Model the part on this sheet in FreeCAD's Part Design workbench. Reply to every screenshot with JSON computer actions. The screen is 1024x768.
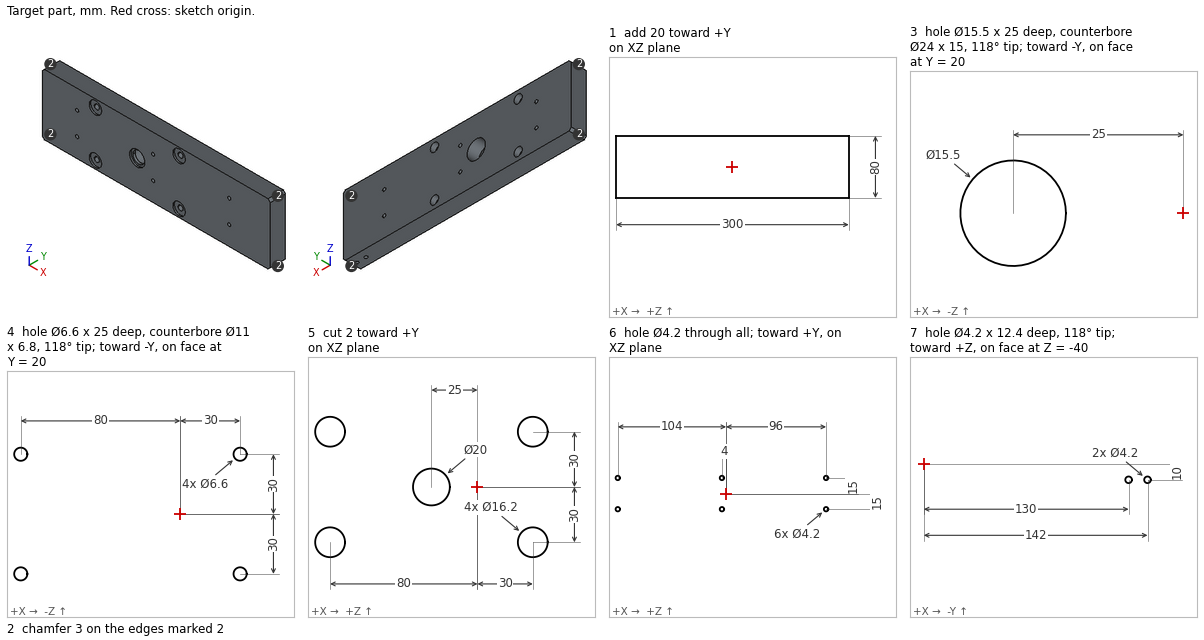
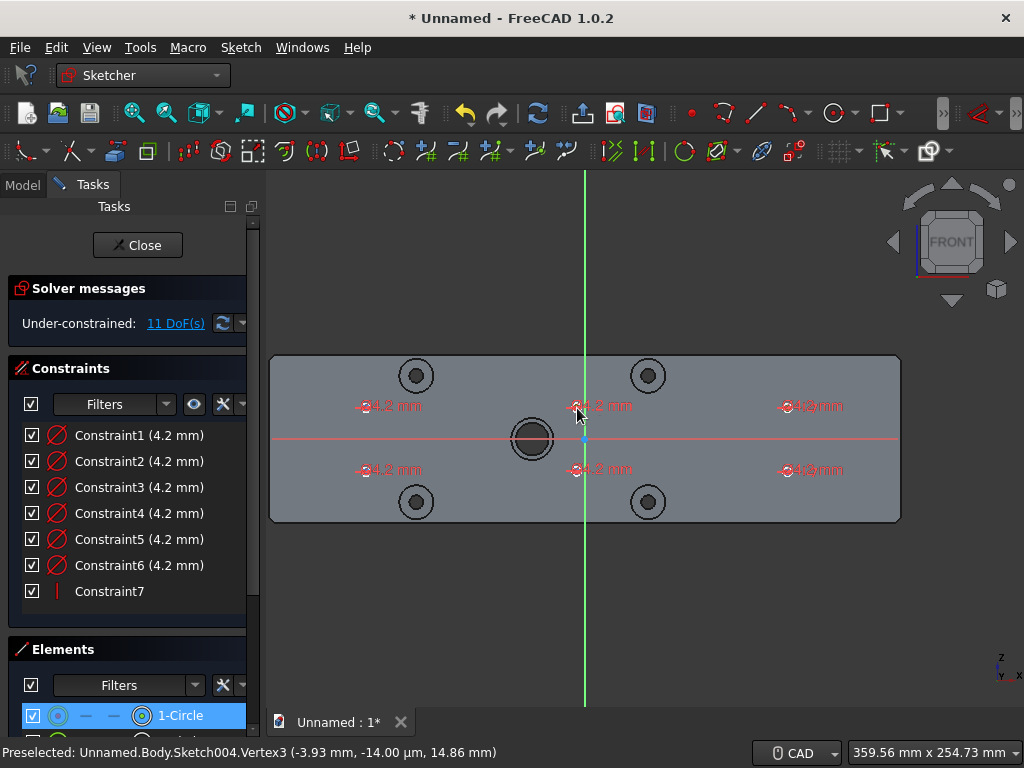
{"action": "key", "text": "h"}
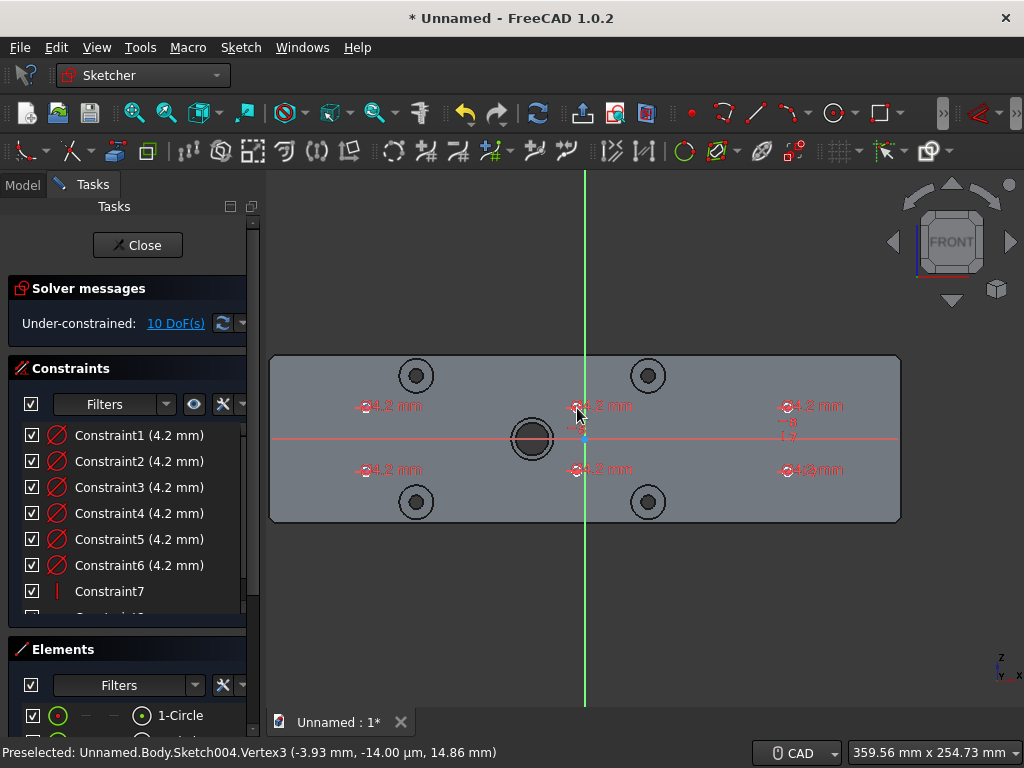
{"action": "left_click", "coordinate": [577, 408]}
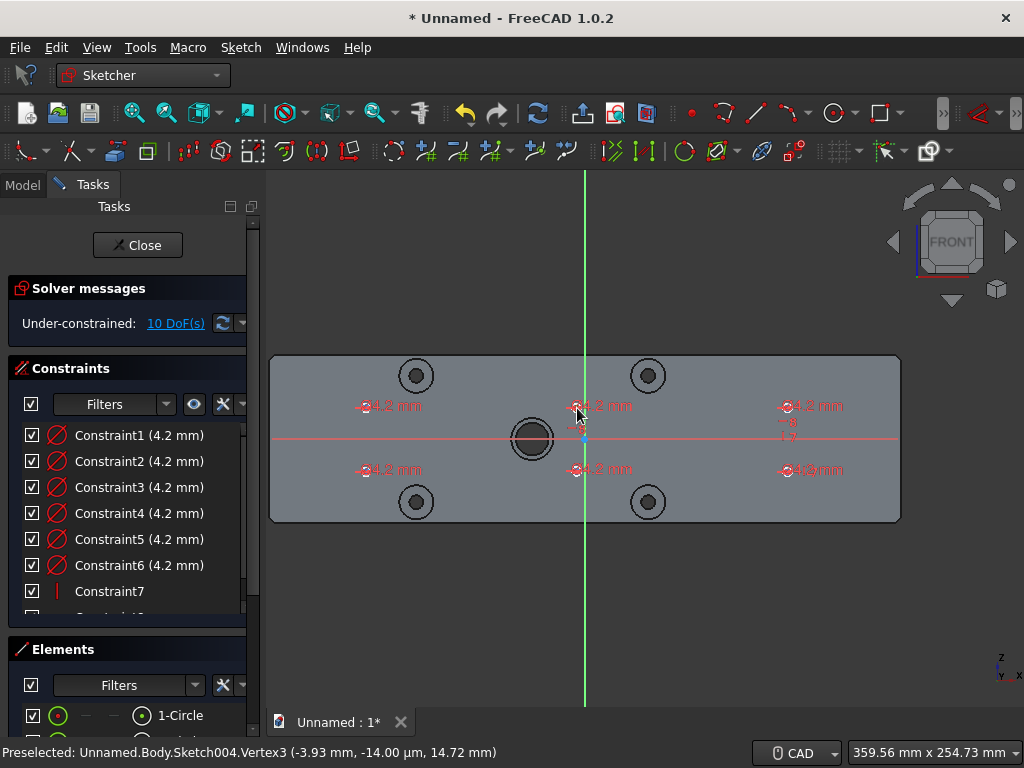
{"action": "left_click", "coordinate": [577, 471]}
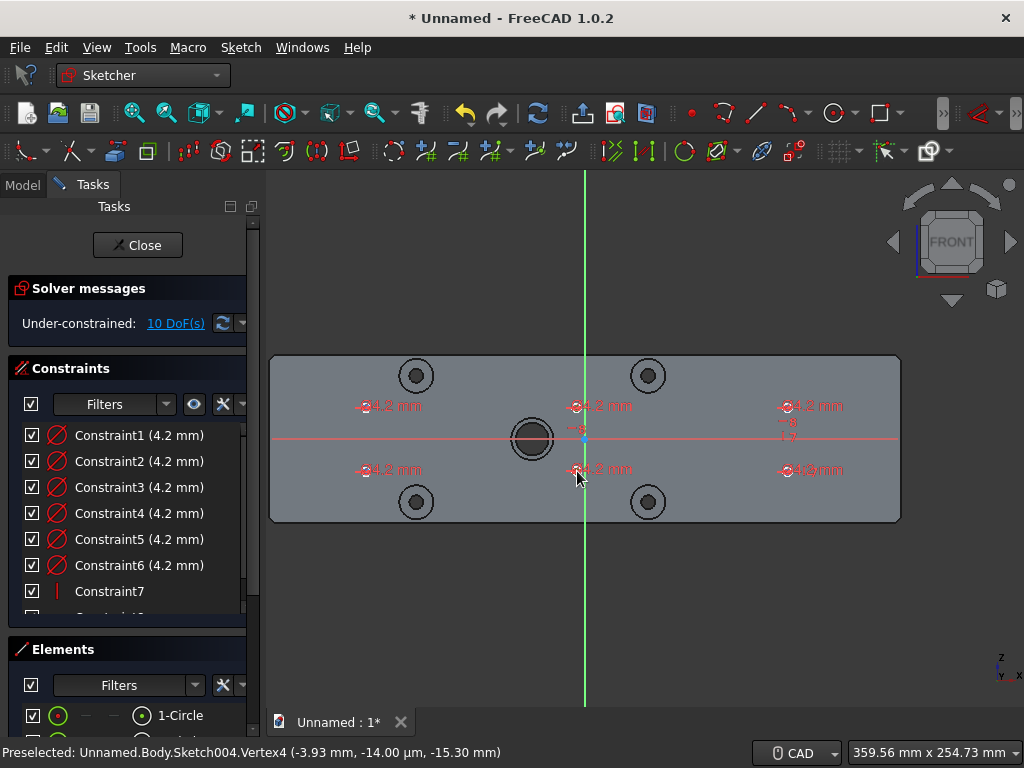
{"action": "key", "text": "v"}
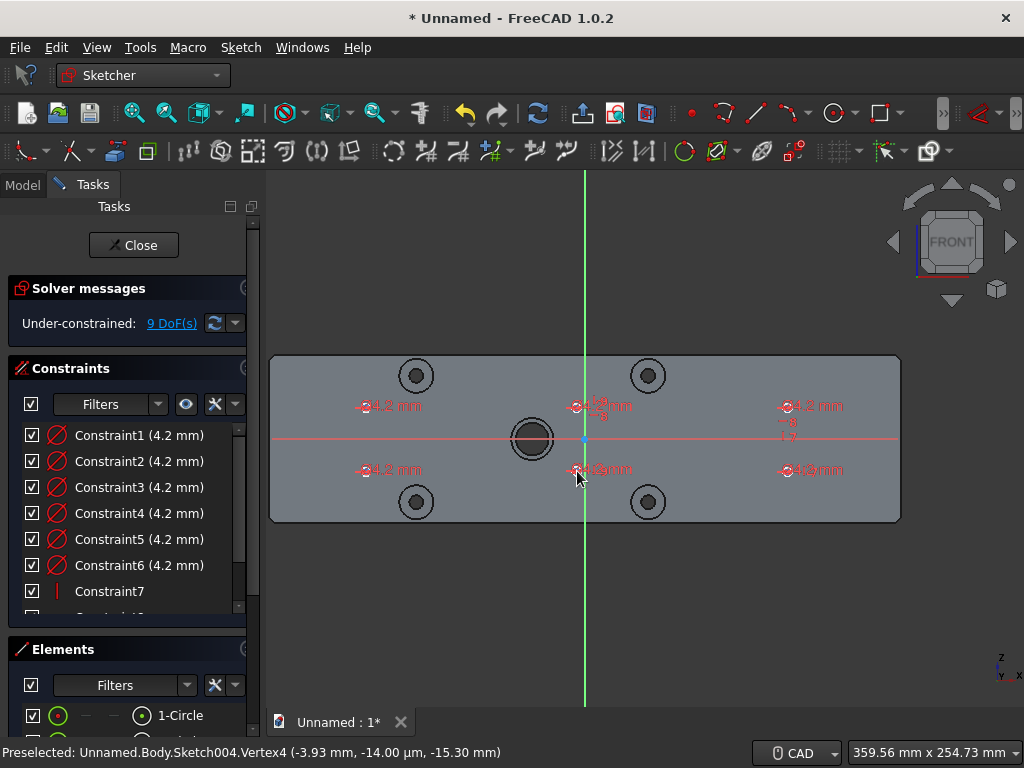
{"action": "left_click", "coordinate": [787, 472]}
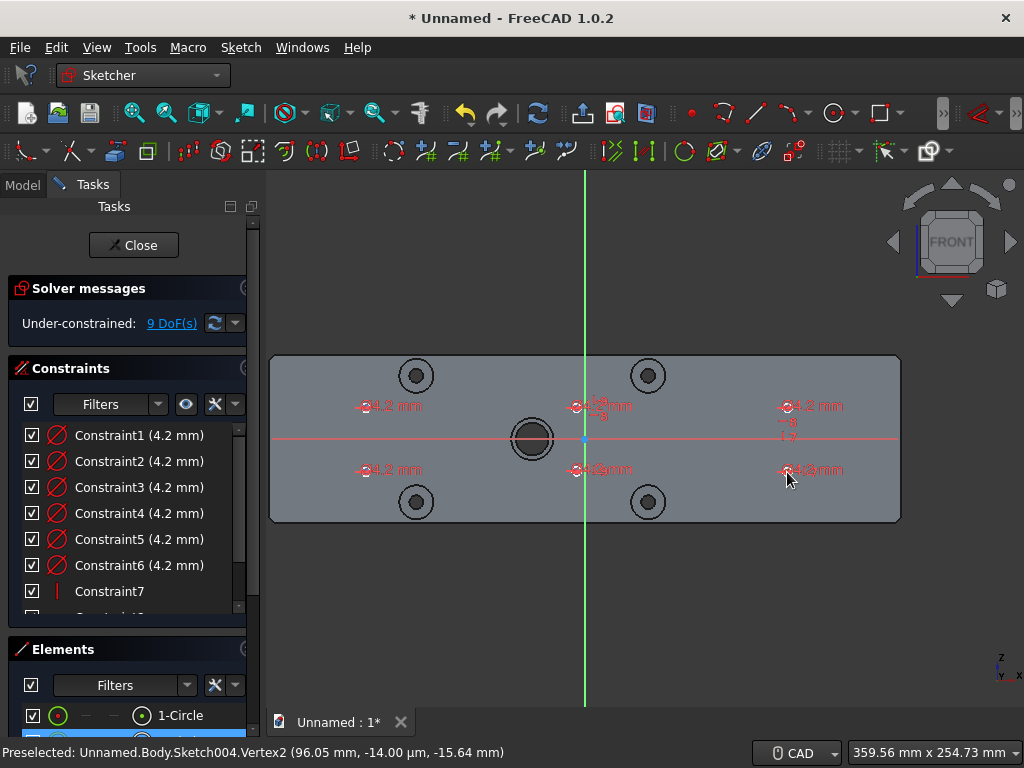
{"action": "left_click", "coordinate": [577, 471]}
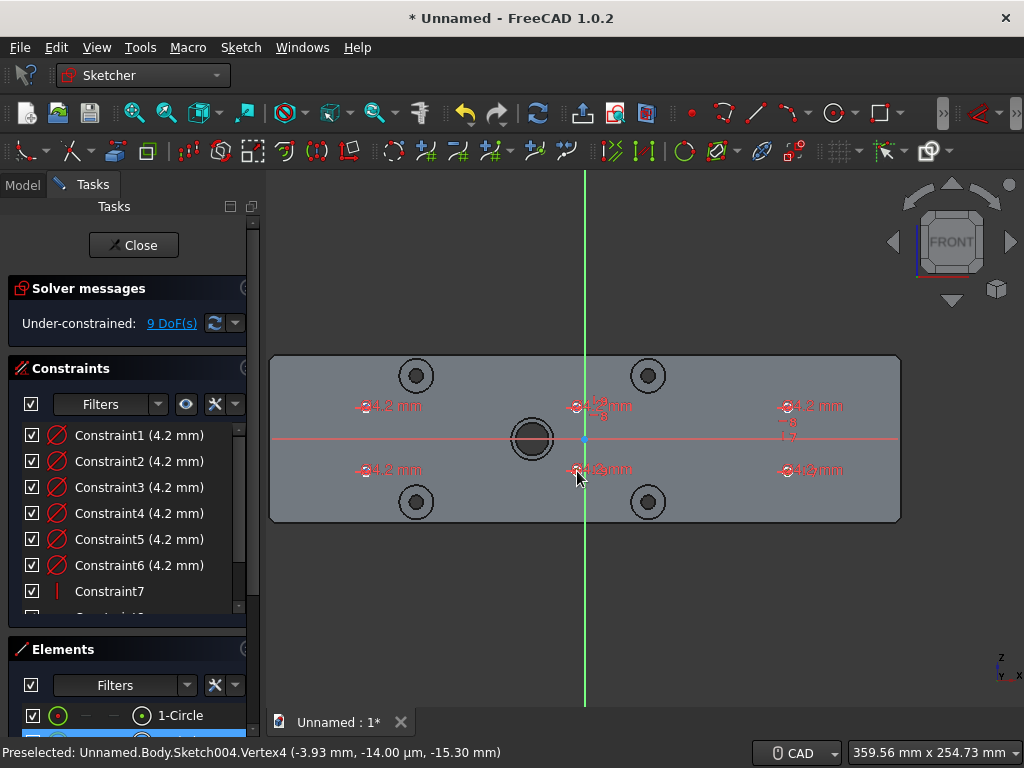
{"action": "key", "text": "h"}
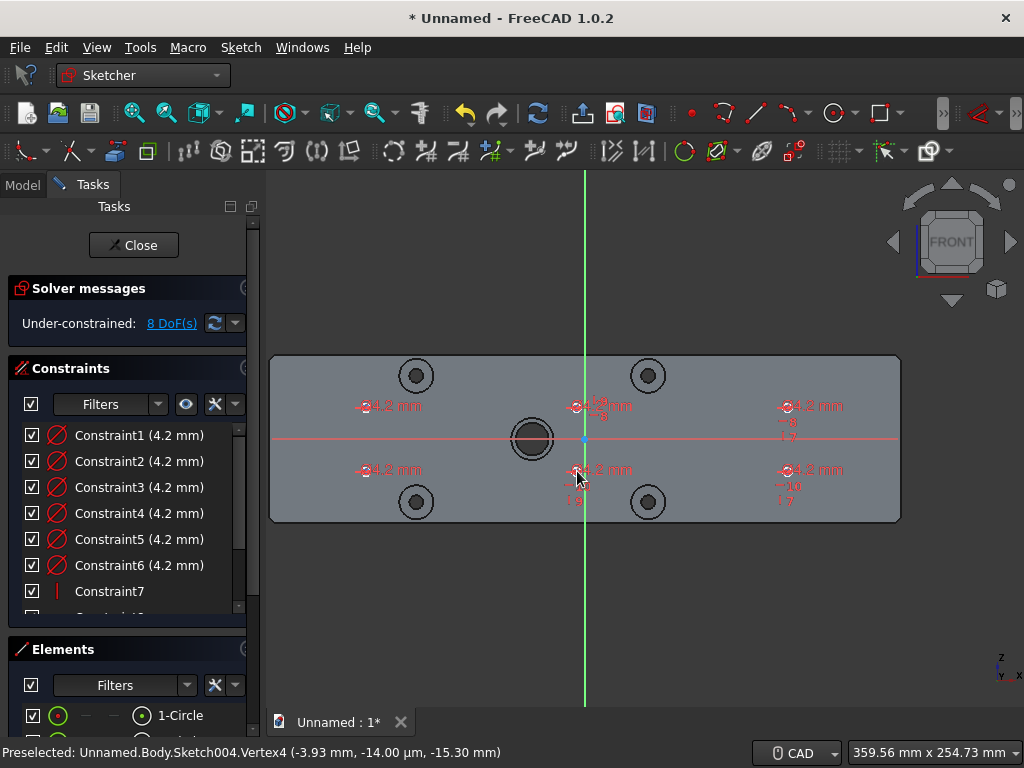
{"action": "left_click", "coordinate": [577, 408]}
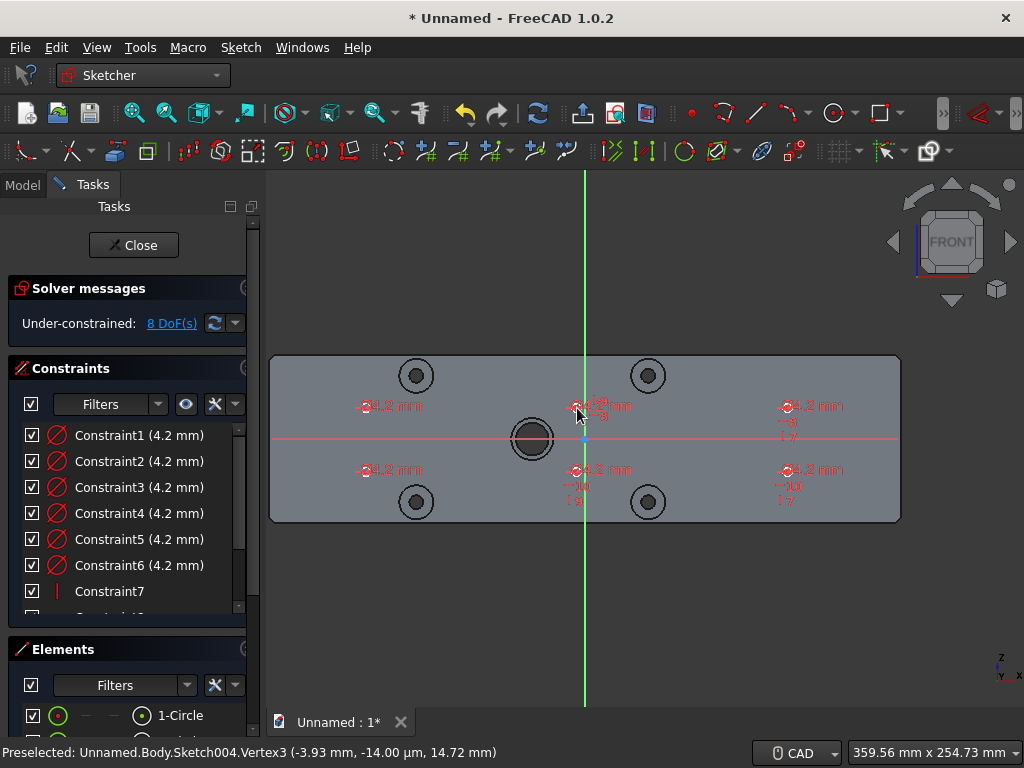
{"action": "left_click", "coordinate": [366, 408]}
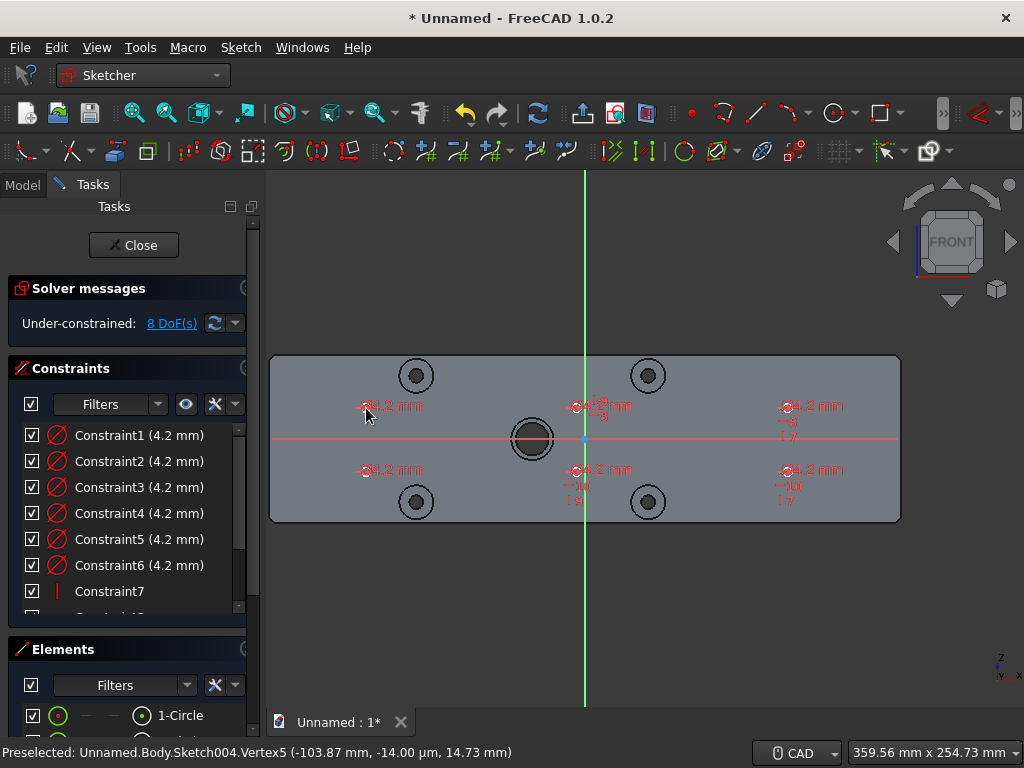
{"action": "key", "text": "h"}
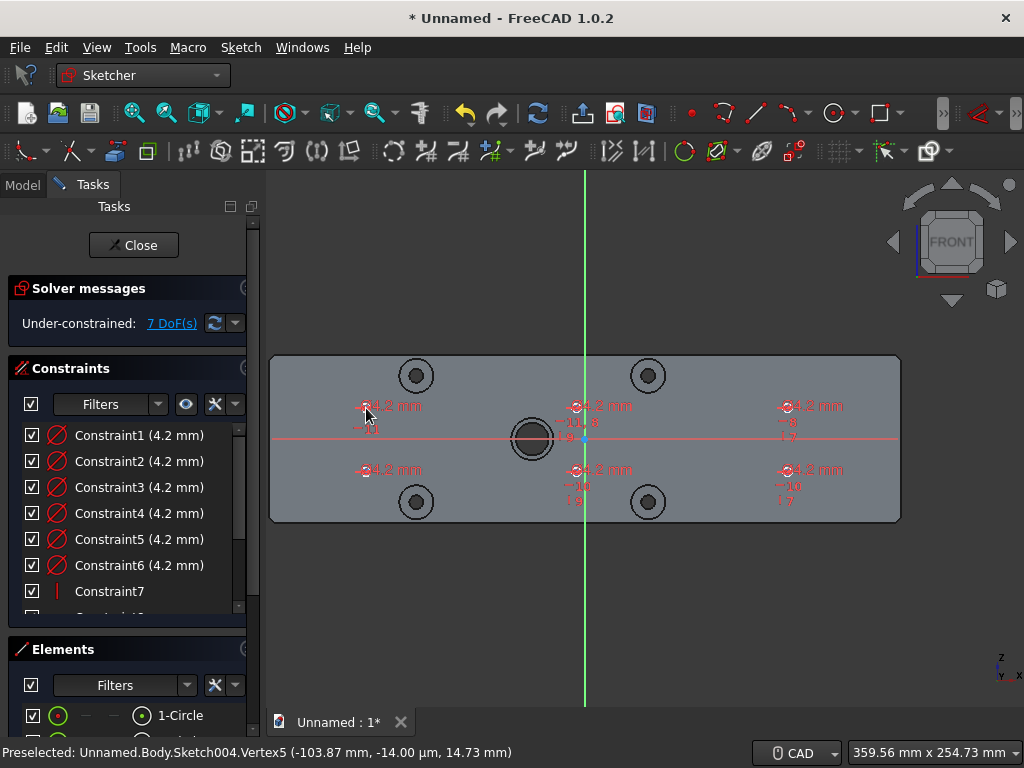
{"action": "left_click", "coordinate": [366, 408]}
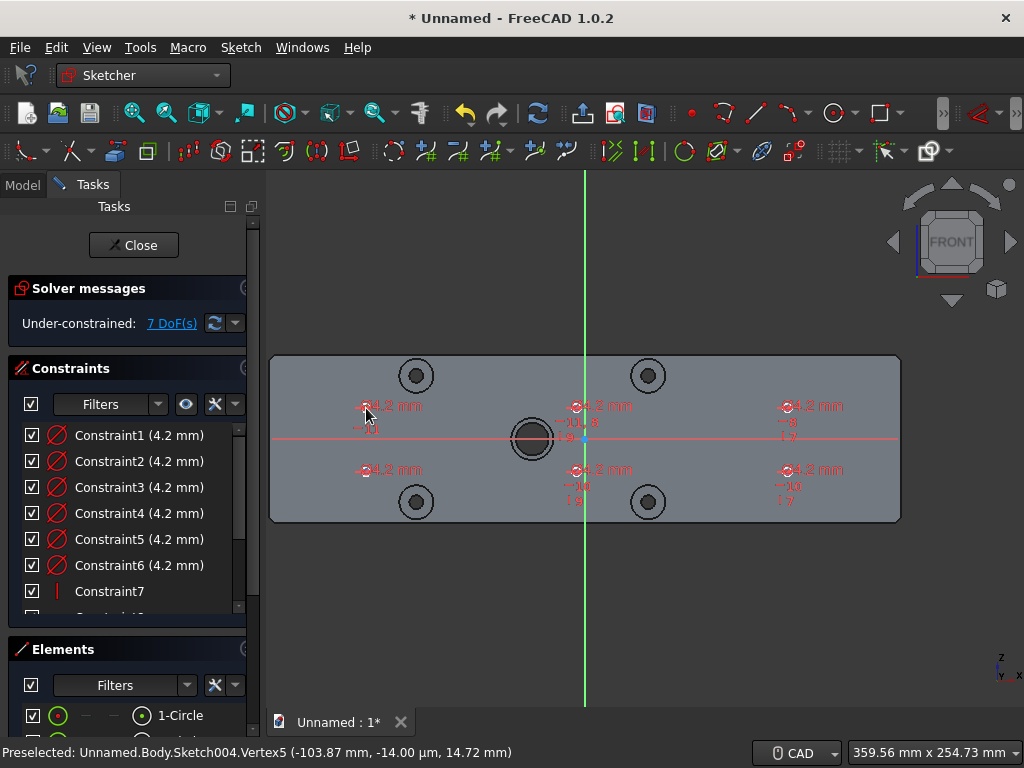
{"action": "left_click", "coordinate": [366, 472]}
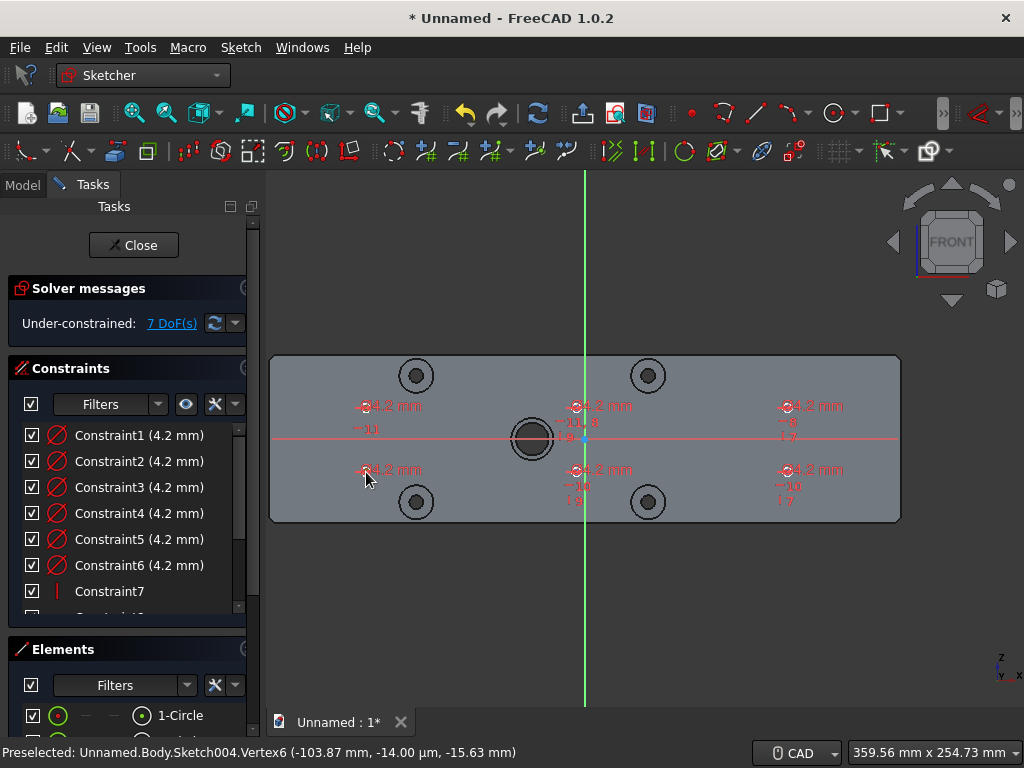
{"action": "key", "text": "v"}